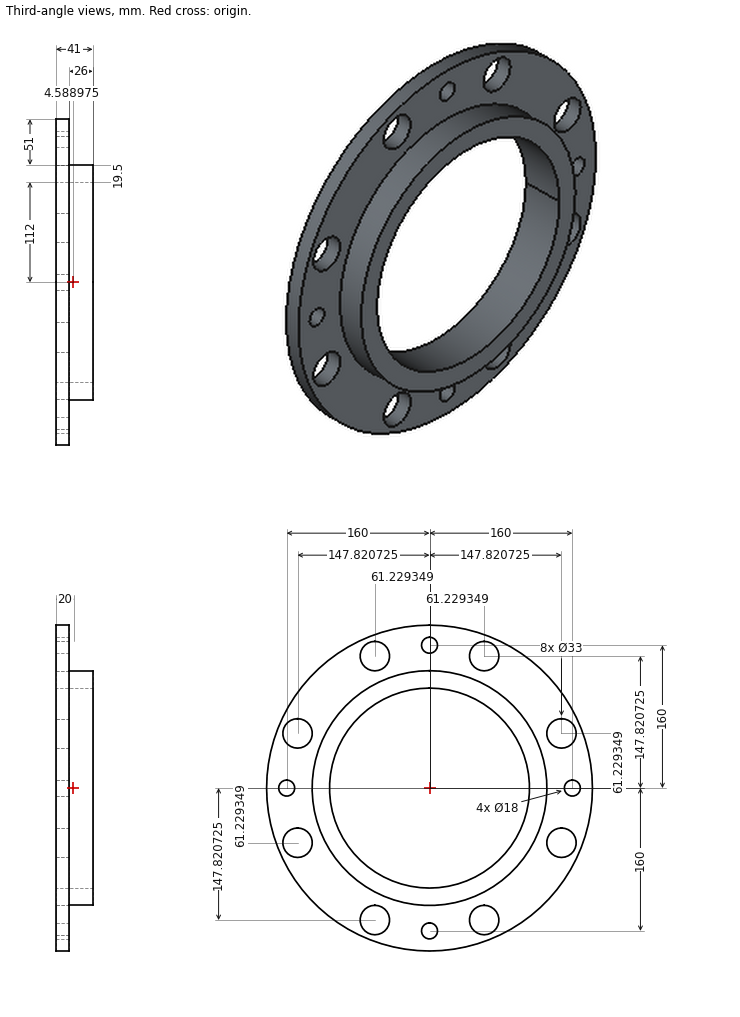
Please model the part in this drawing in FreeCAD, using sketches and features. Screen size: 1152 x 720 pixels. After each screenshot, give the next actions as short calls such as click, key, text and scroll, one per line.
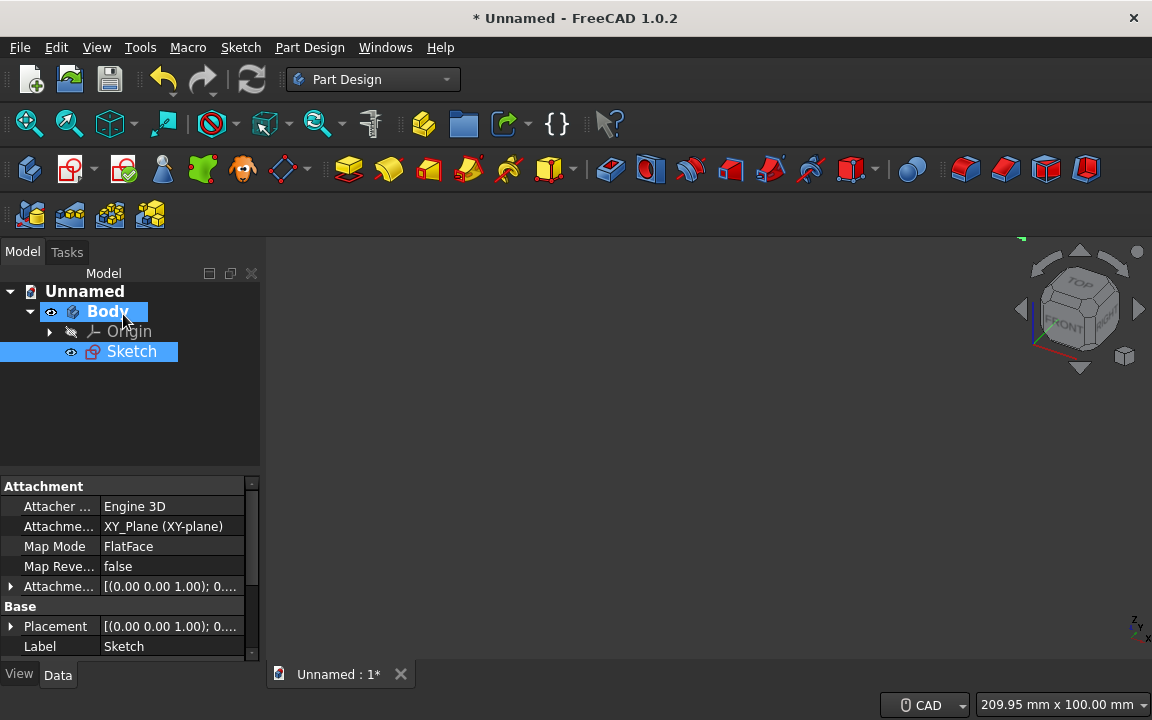
click(390, 170)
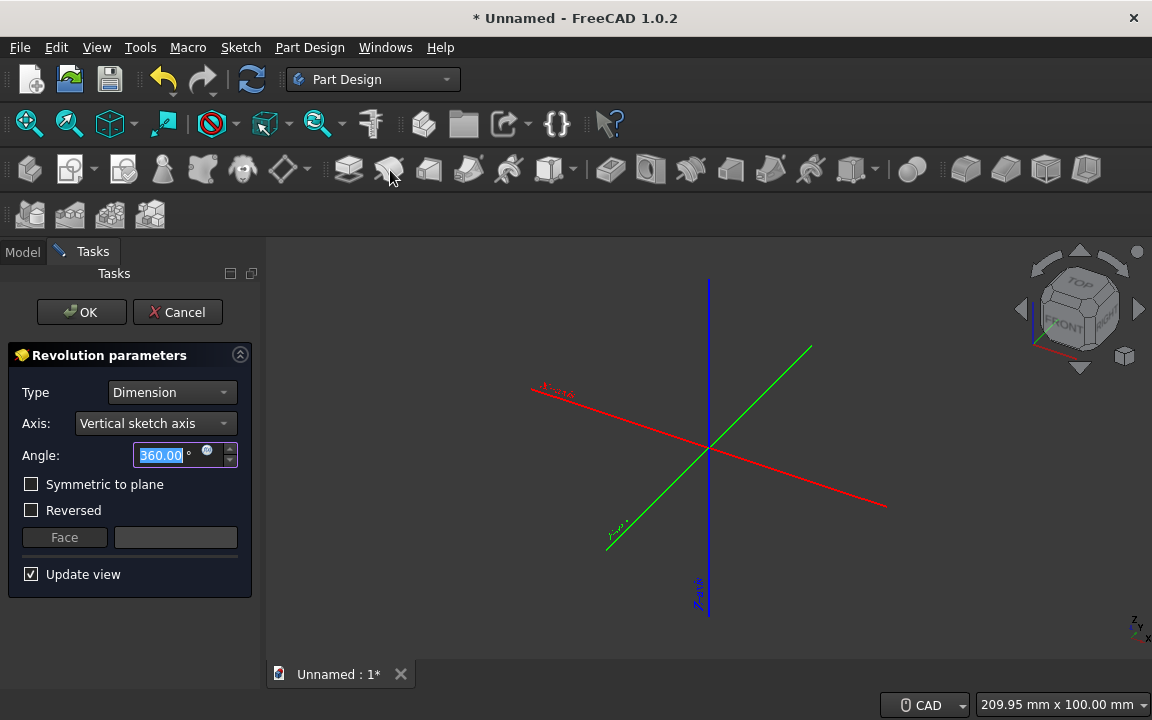
click(156, 424)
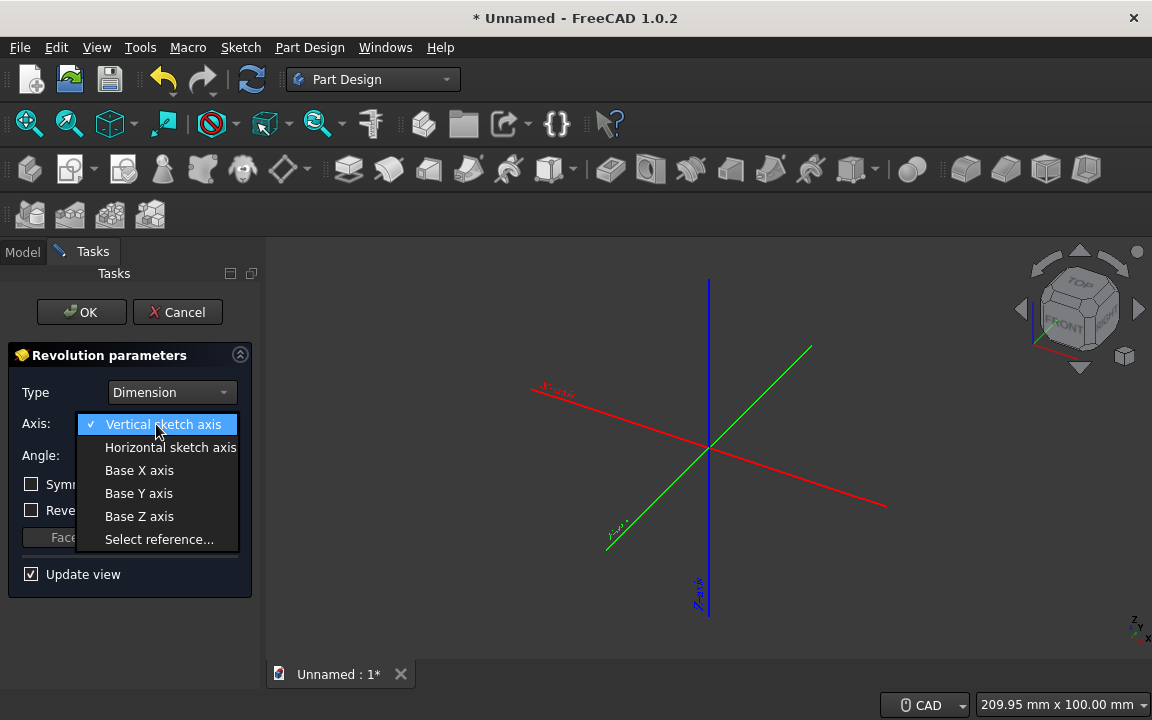
click(156, 448)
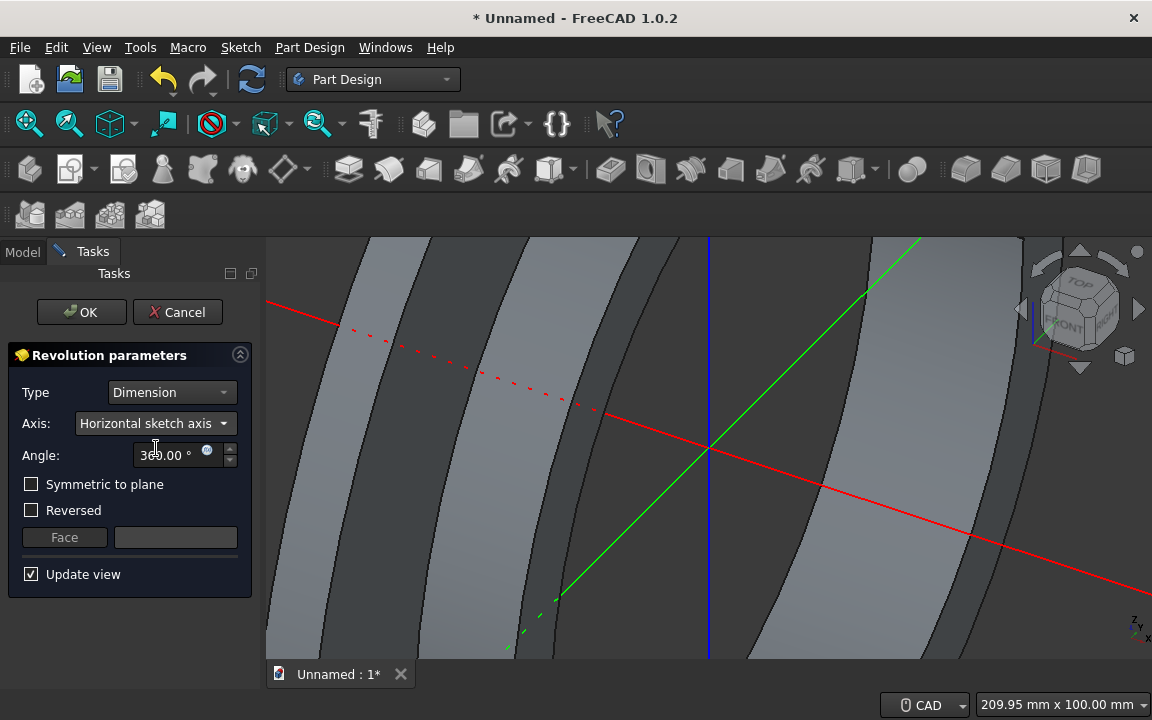
click(82, 312)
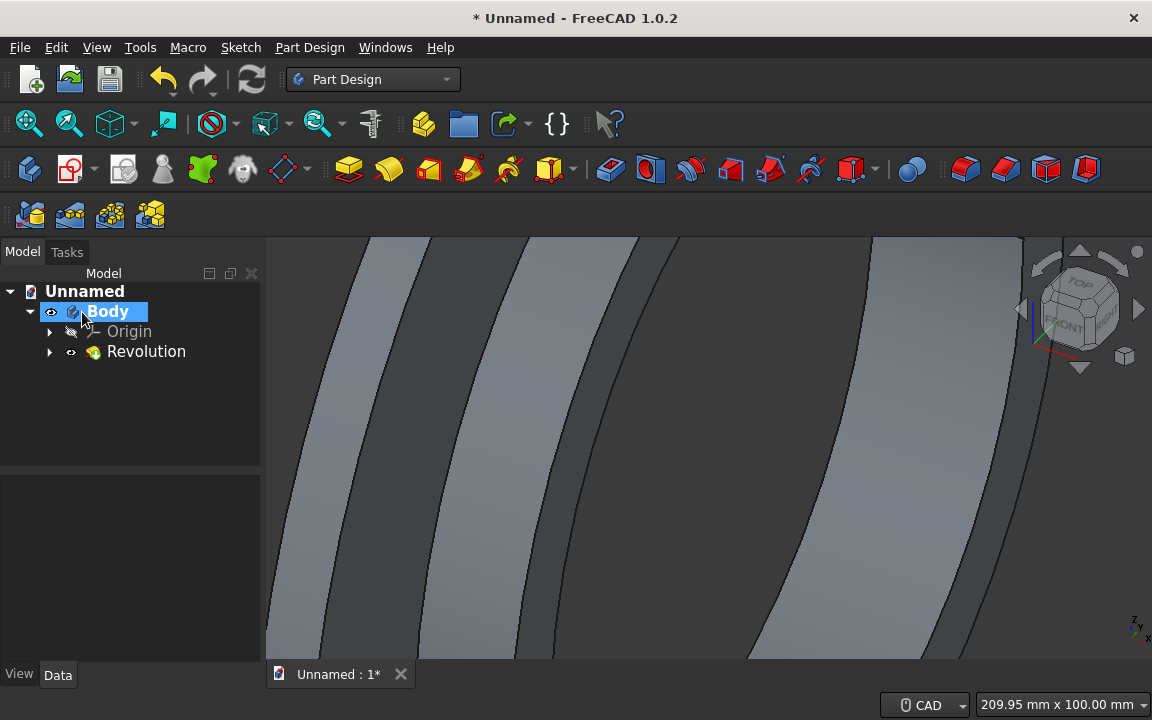
click(30, 124)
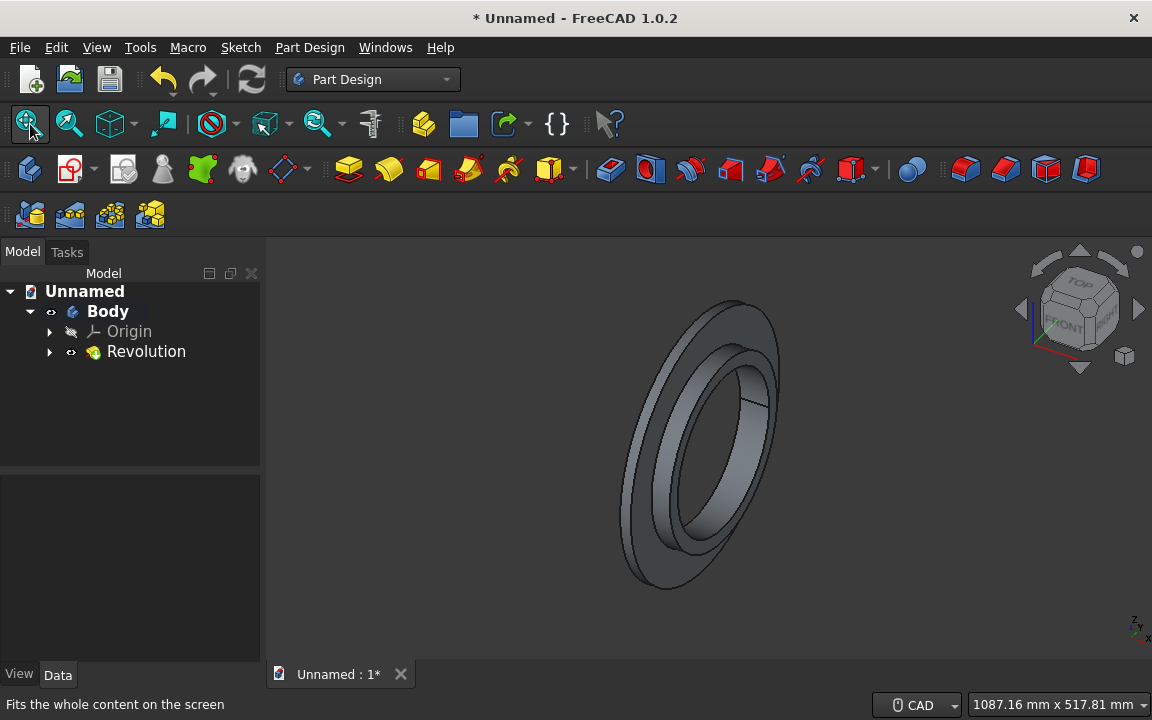
key(6)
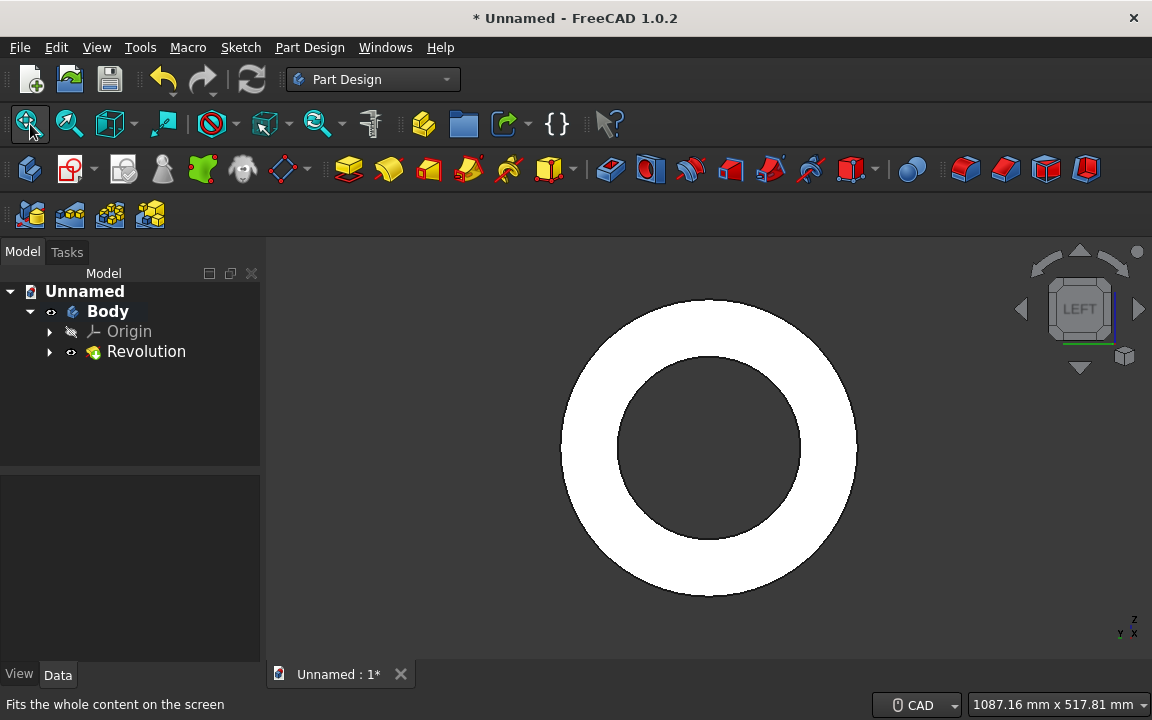
click(624, 362)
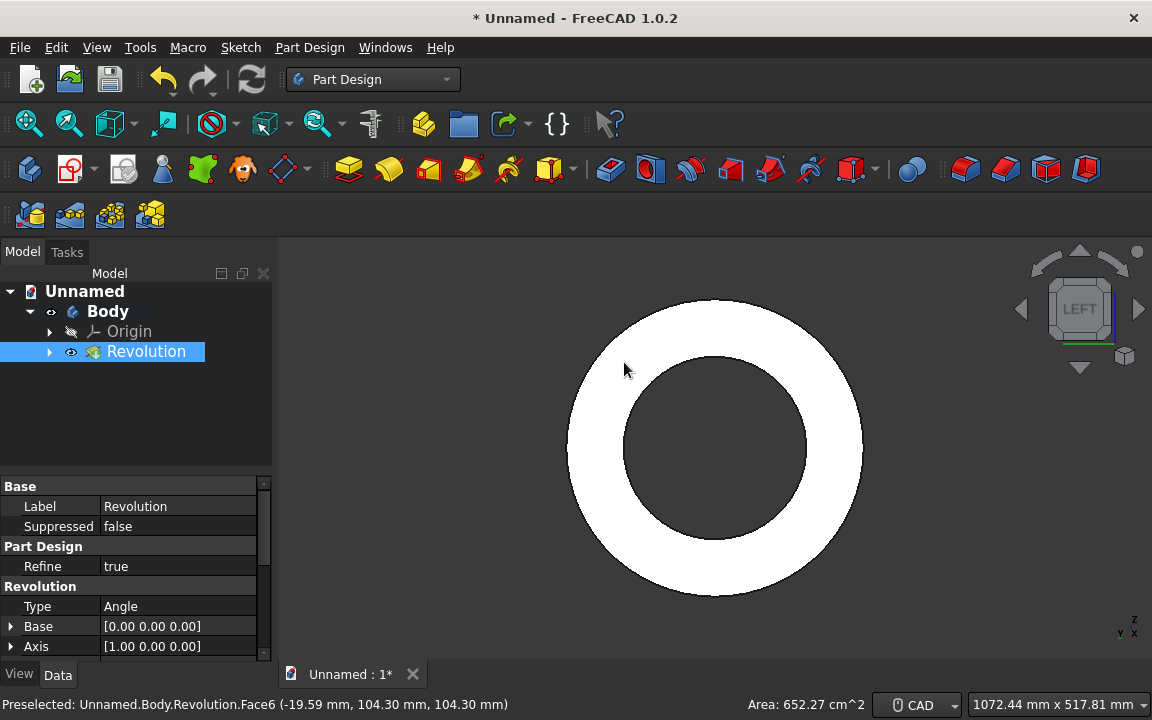
click(70, 170)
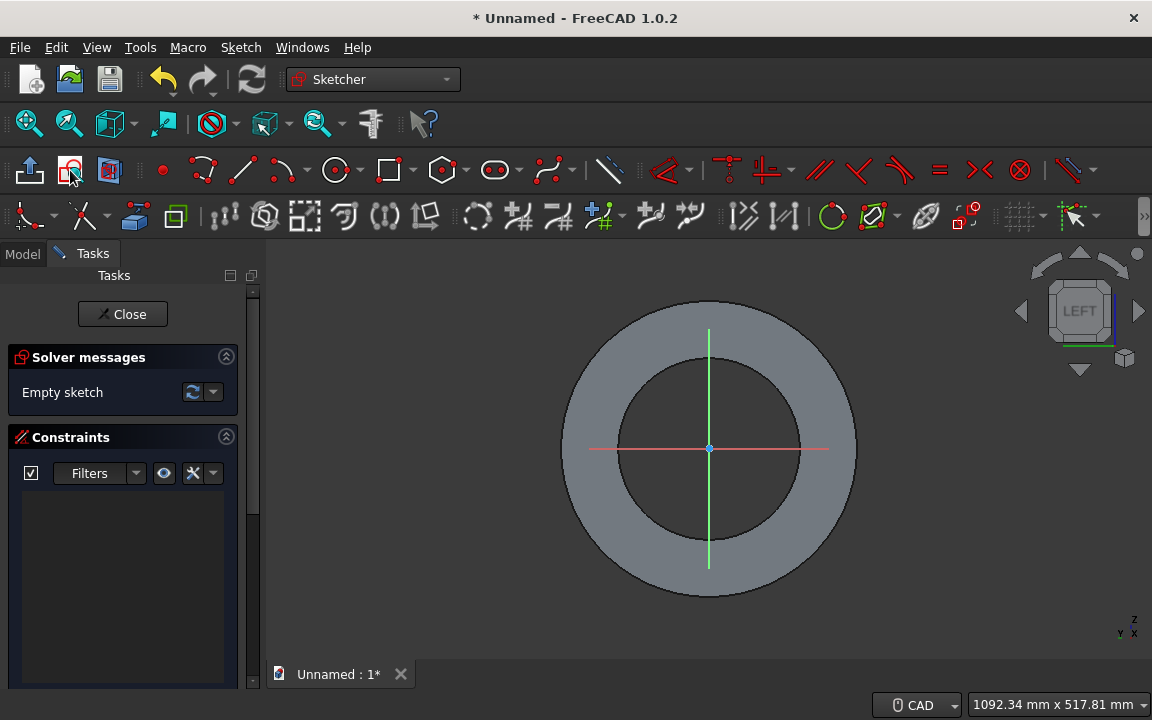
click(336, 170)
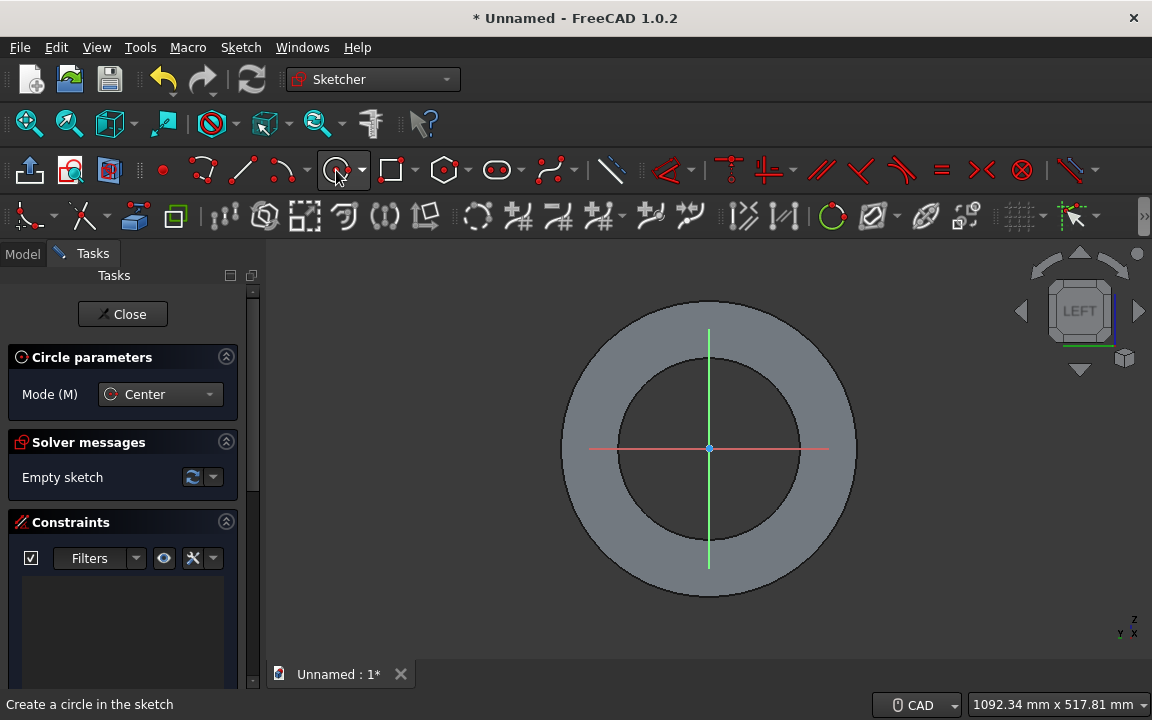
scroll(589, 399, up, 3)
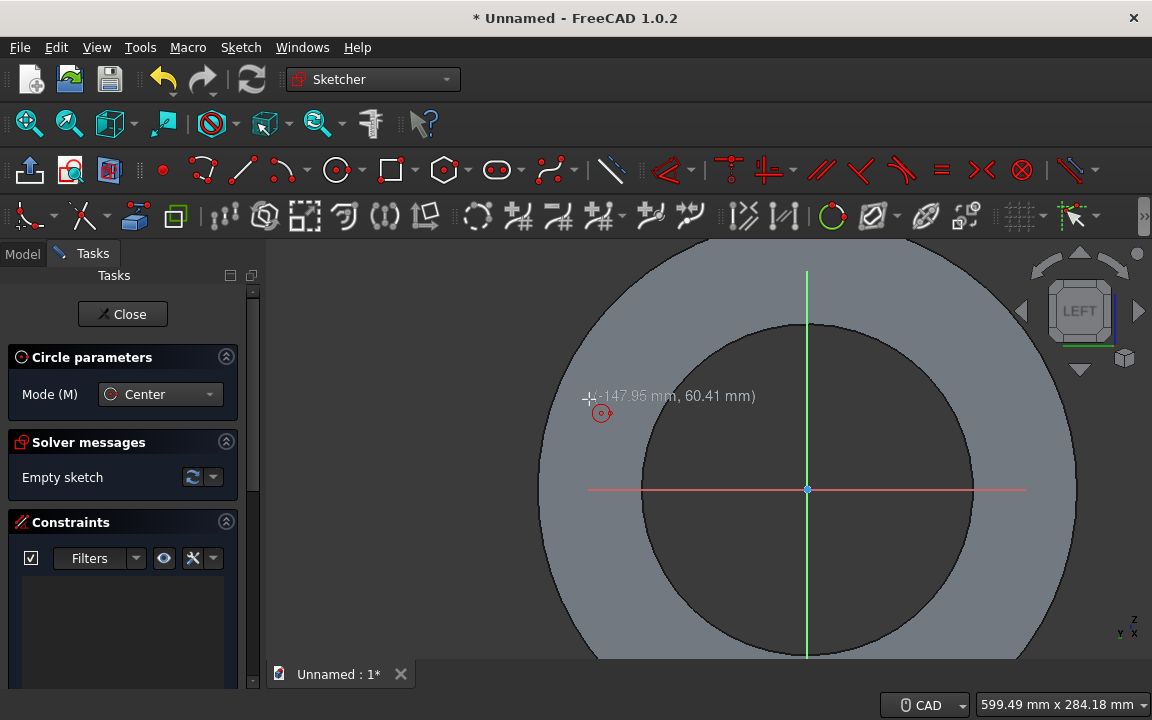
click(589, 399)
click(606, 382)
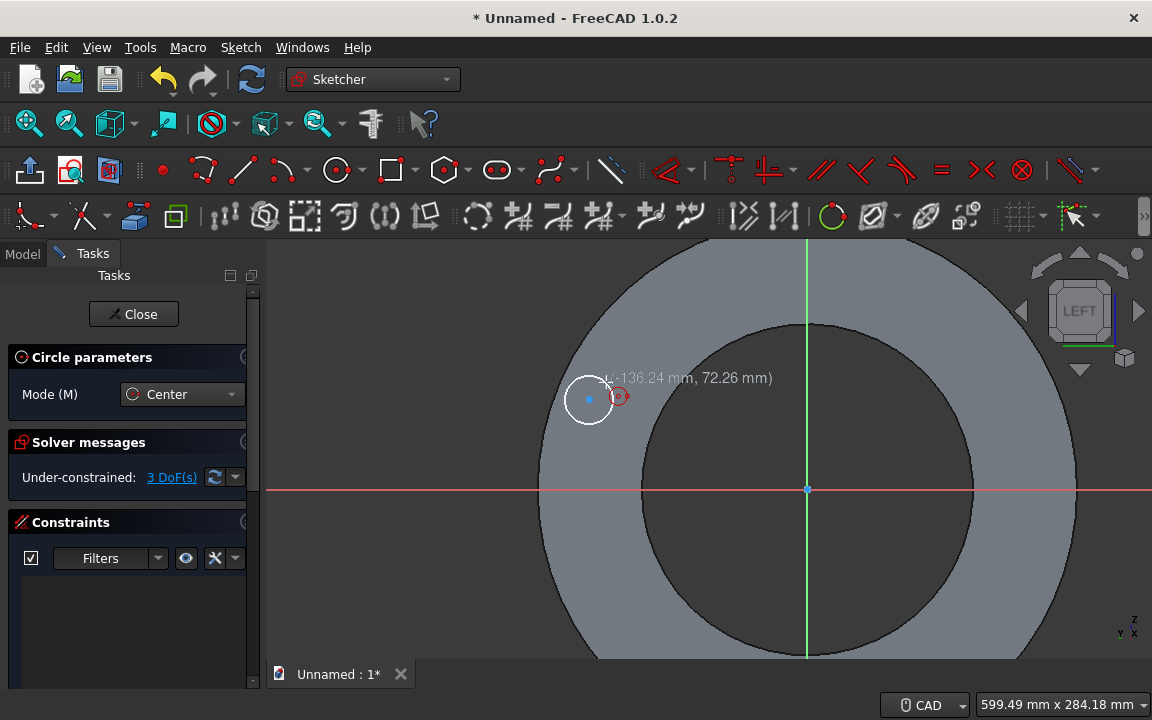
click(717, 271)